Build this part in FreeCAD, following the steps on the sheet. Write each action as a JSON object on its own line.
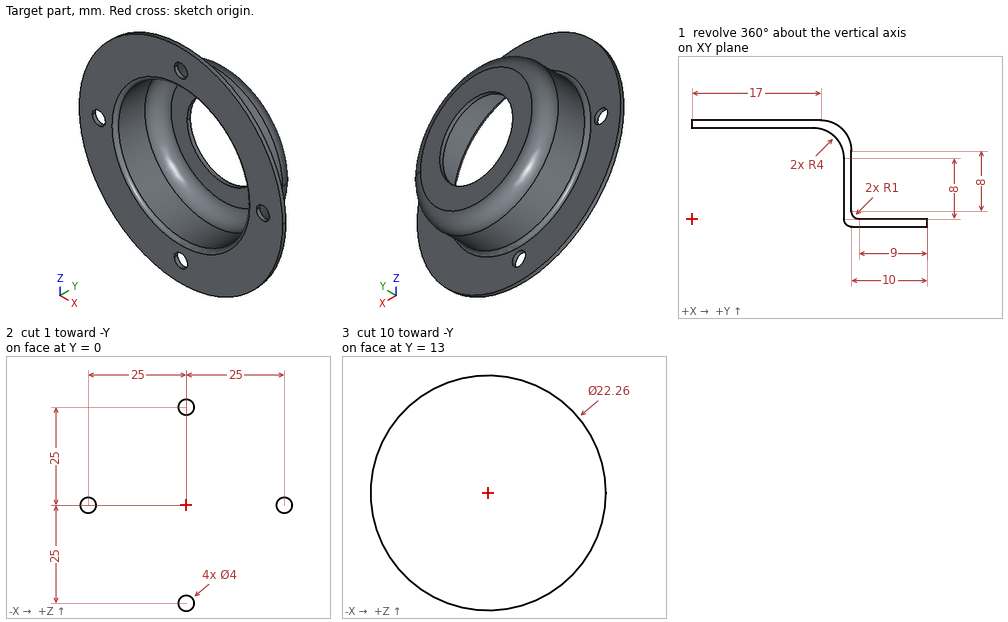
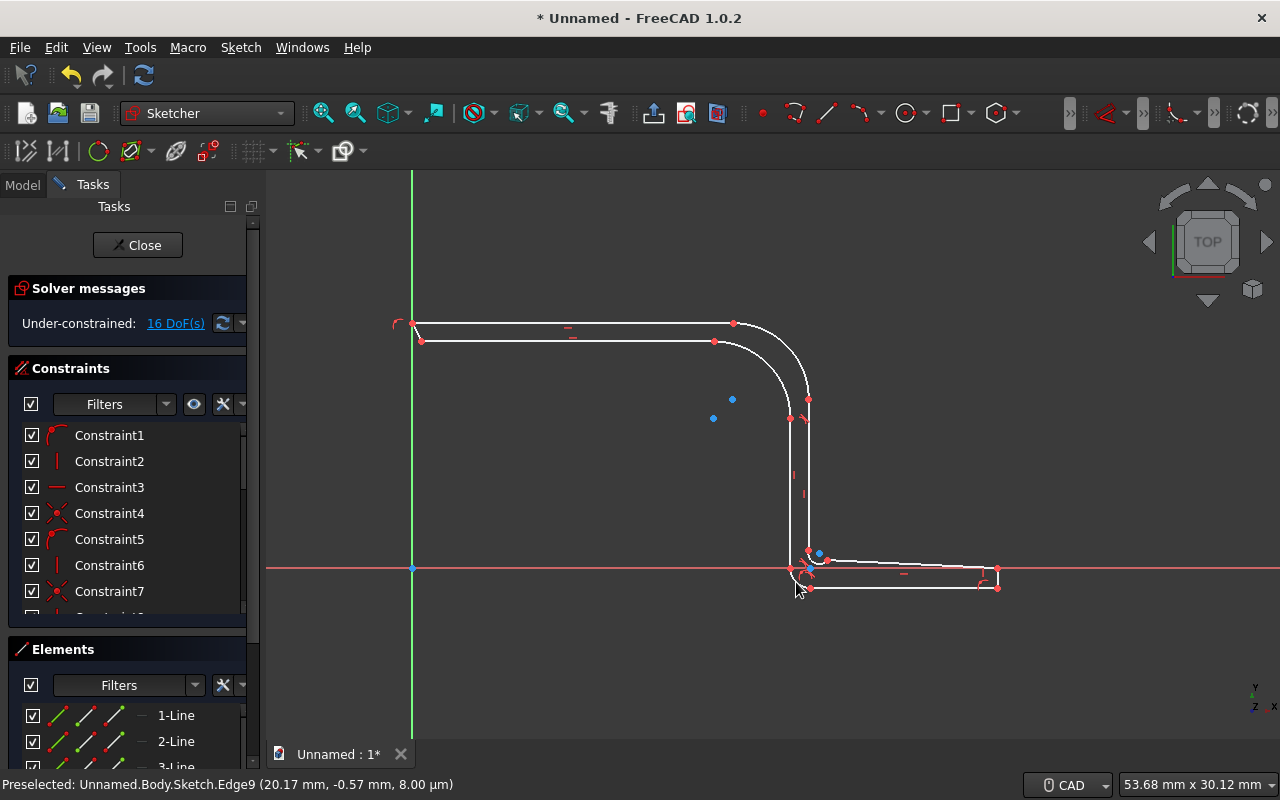
{"action": "left_click", "coordinate": [947, 566]}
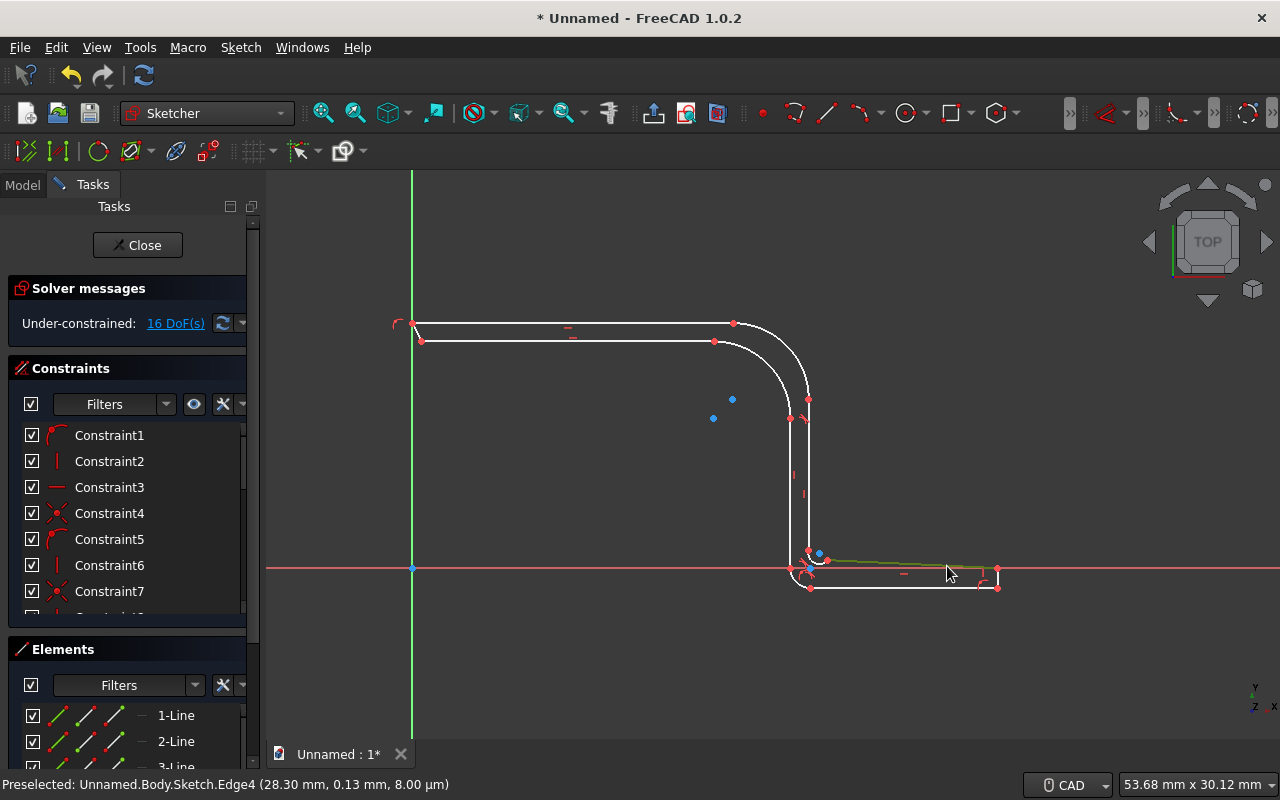
{"action": "scroll", "coordinate": [810, 559], "scroll_direction": "up", "scroll_amount": 3}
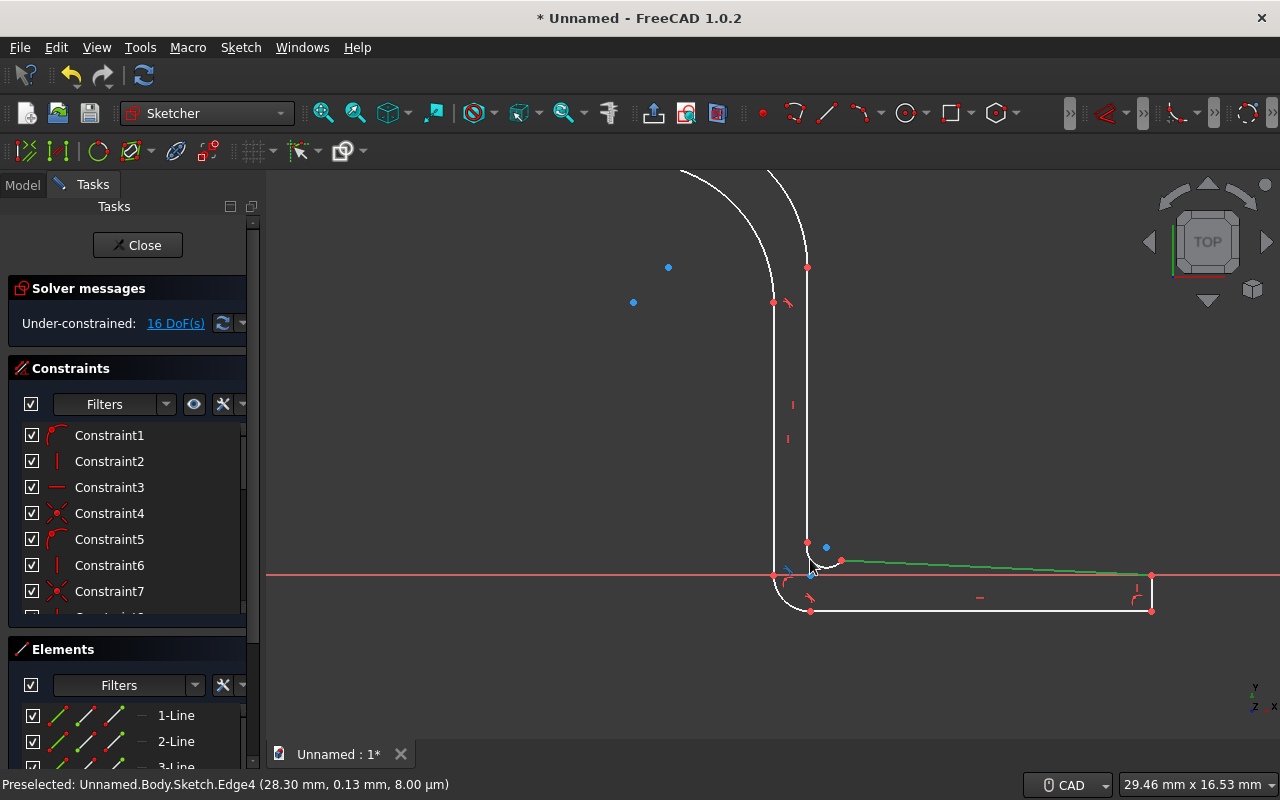
{"action": "left_click", "coordinate": [809, 558]}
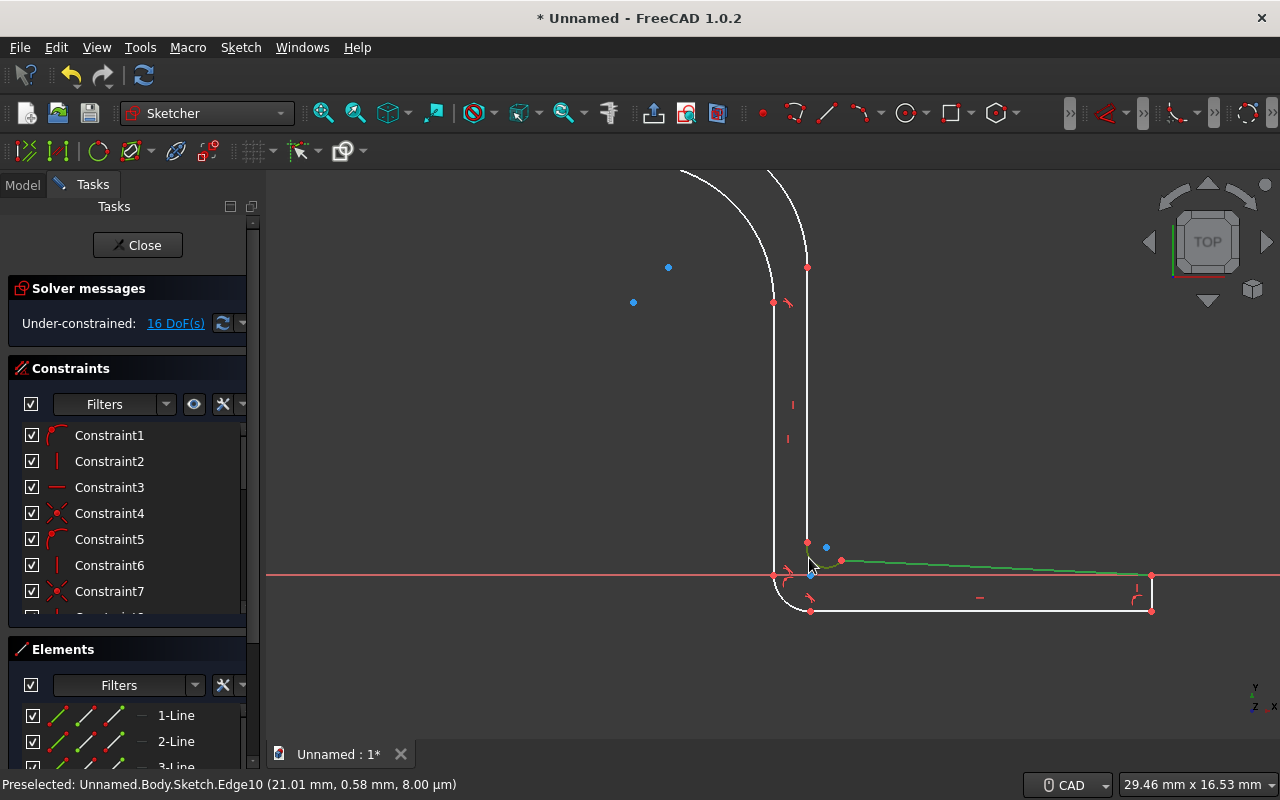
{"action": "key", "text": "t"}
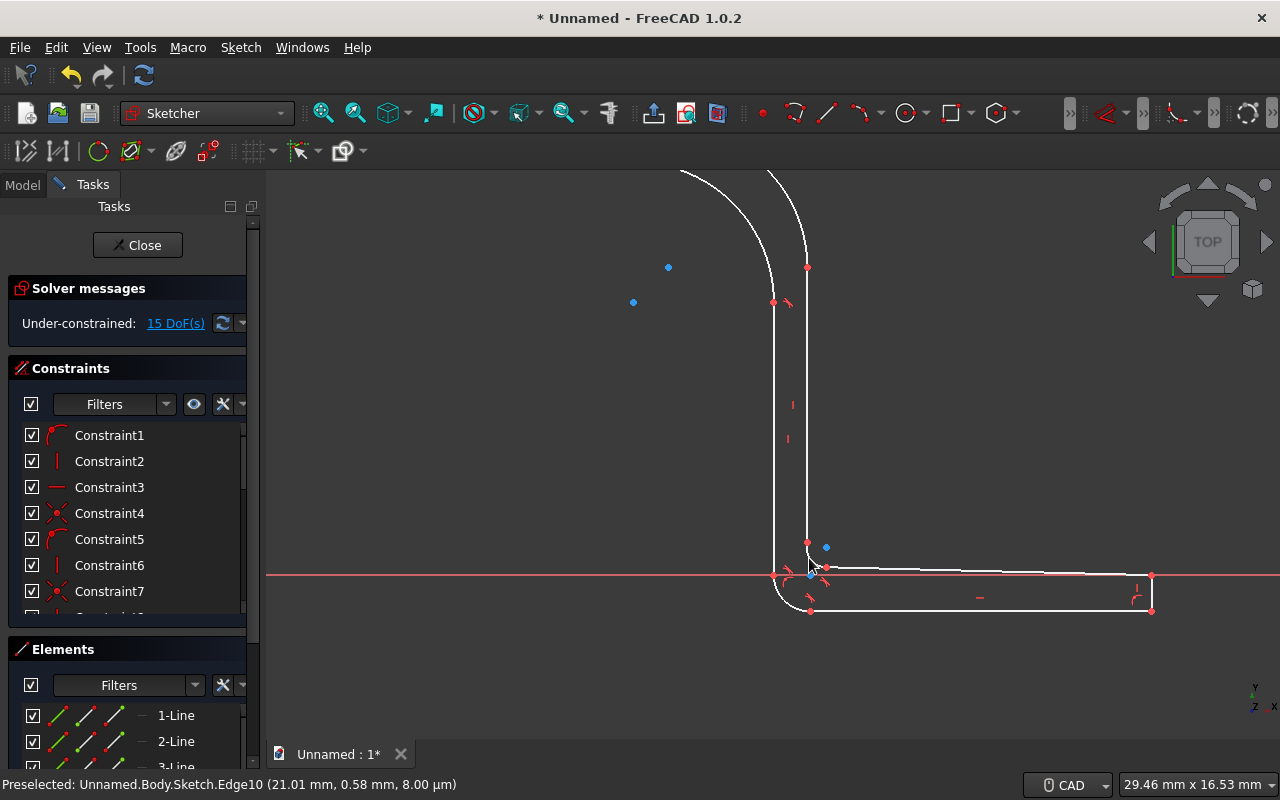
{"action": "left_click", "coordinate": [807, 460]}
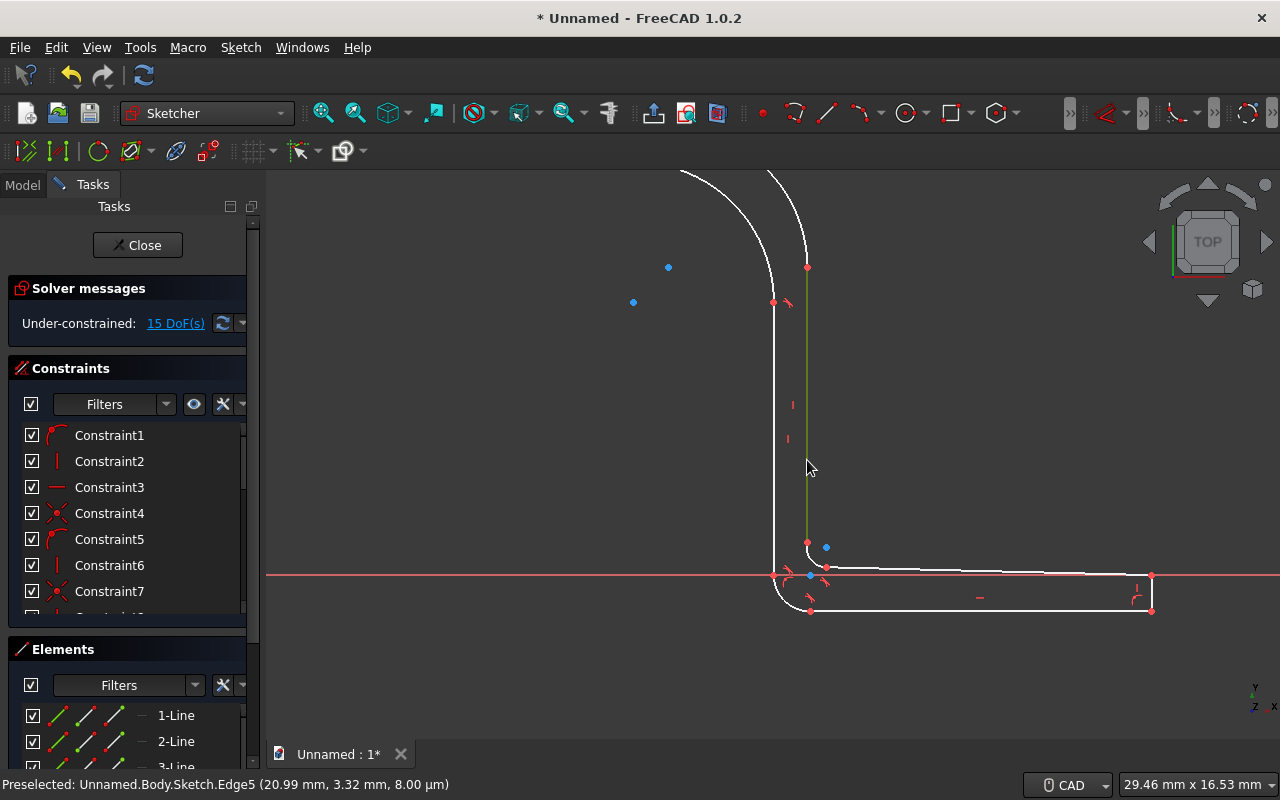
{"action": "scroll", "coordinate": [807, 553], "scroll_direction": "up", "scroll_amount": 2}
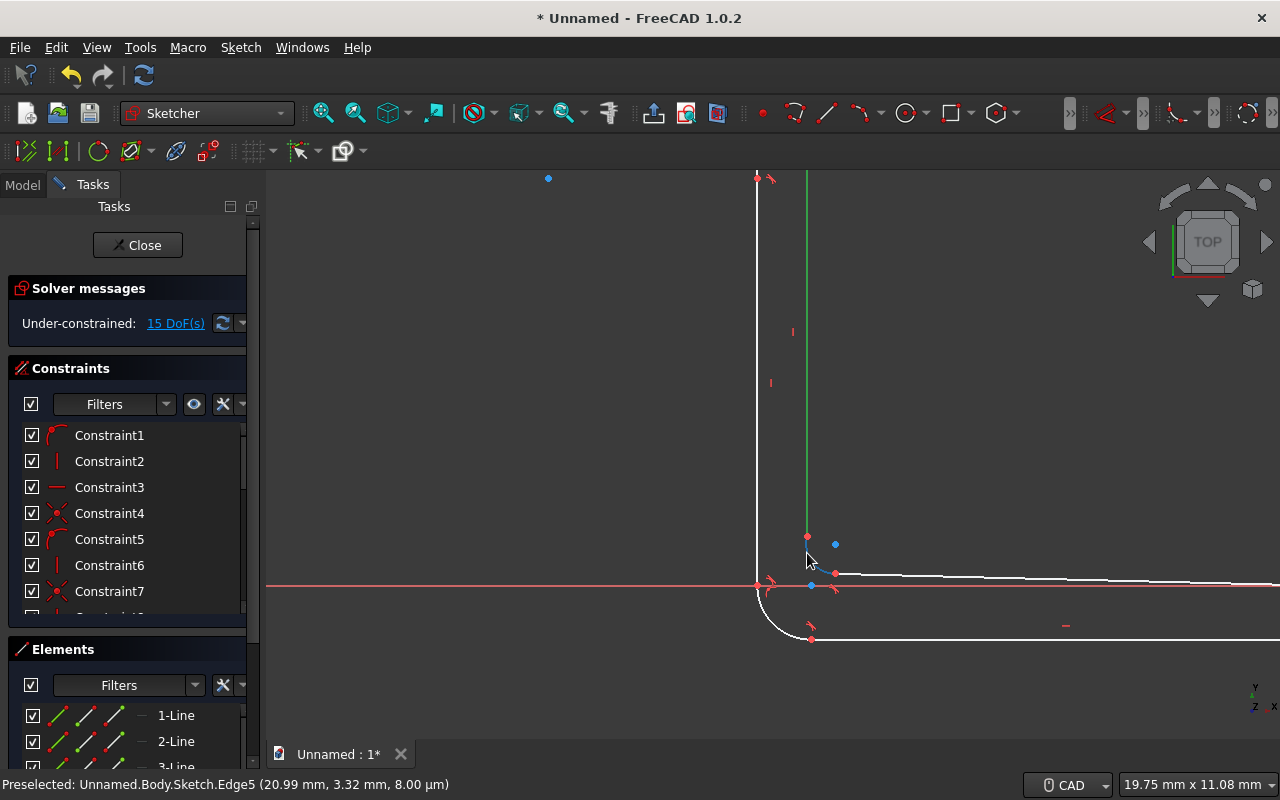
{"action": "left_click", "coordinate": [807, 552]}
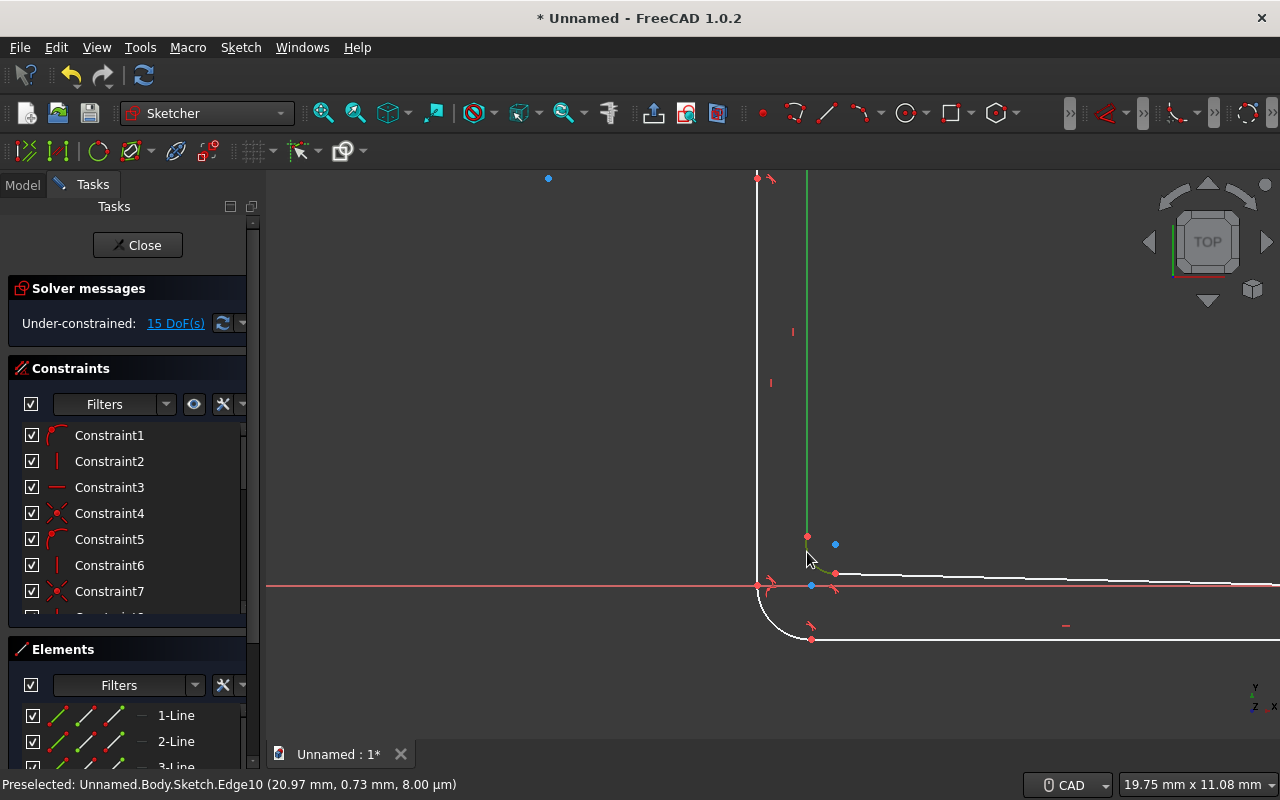
{"action": "key", "text": "t"}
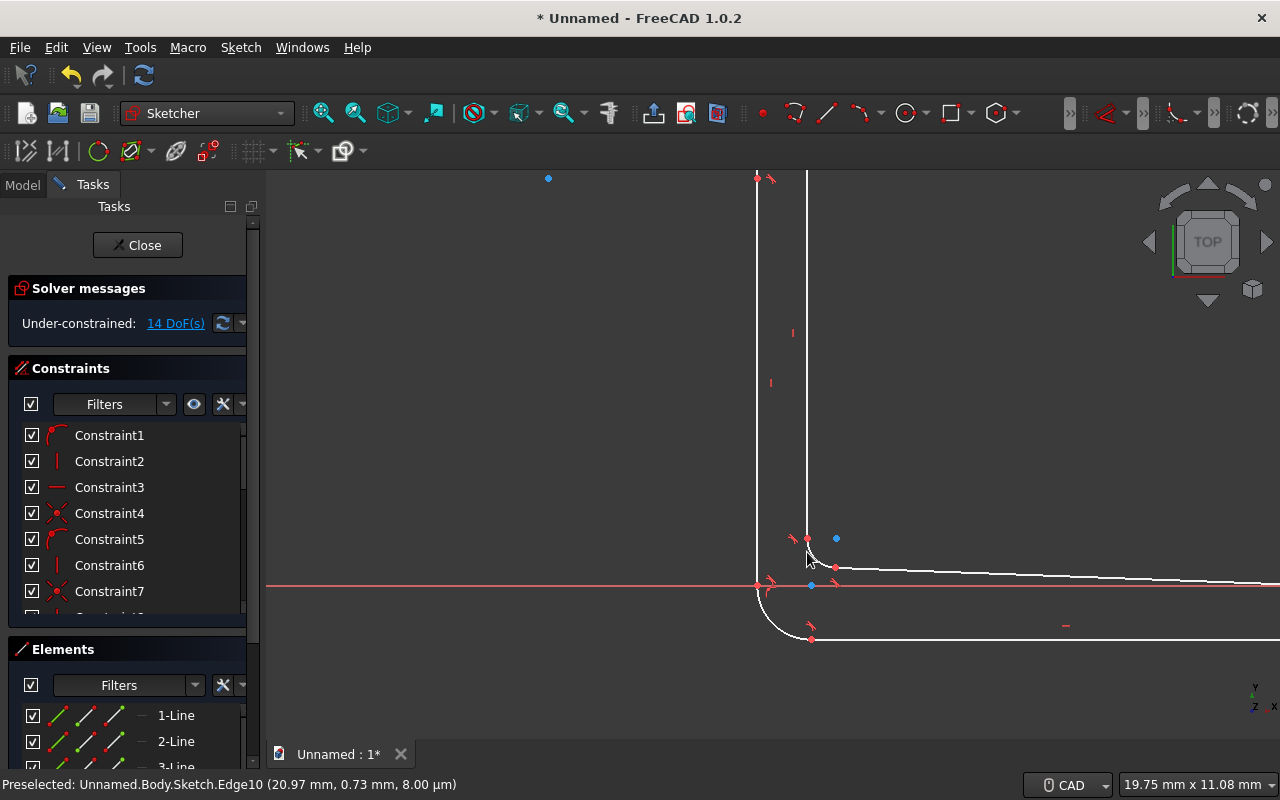
{"action": "left_click", "coordinate": [807, 415]}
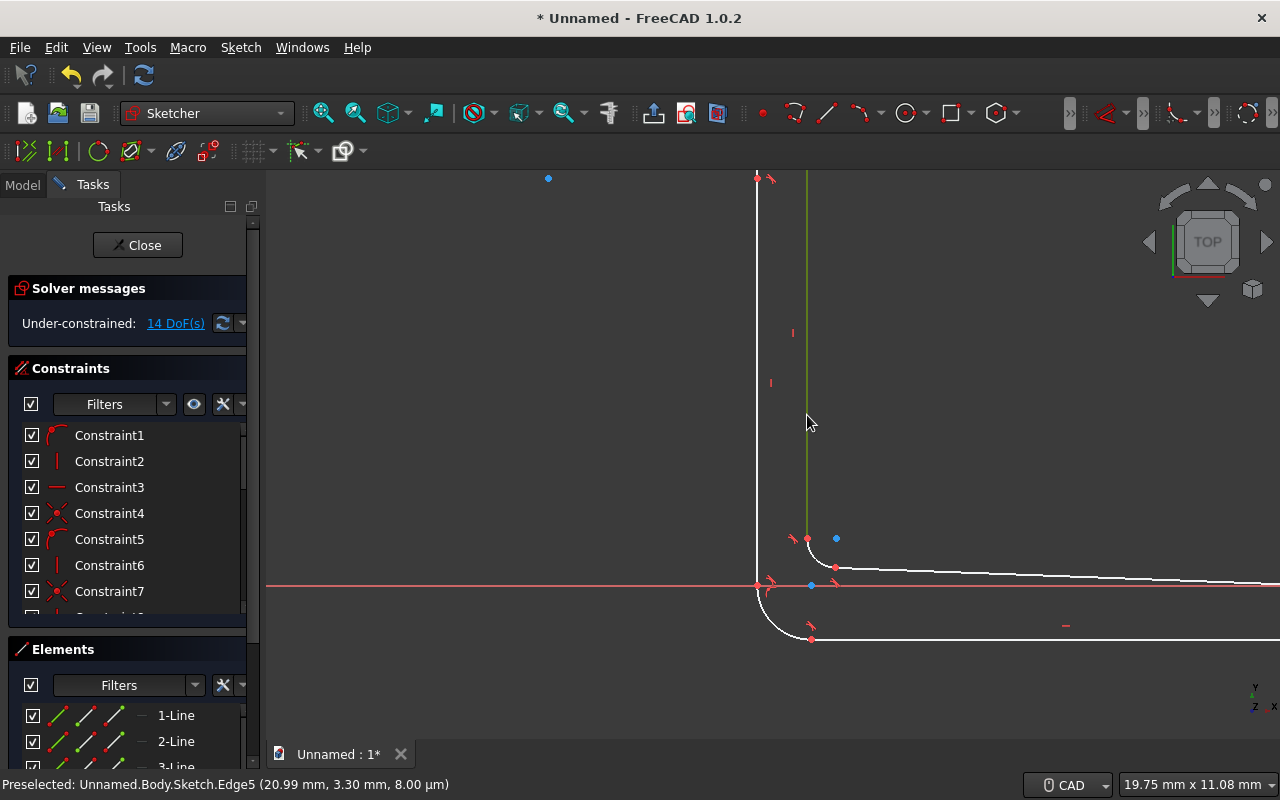
{"action": "scroll", "coordinate": [809, 557], "scroll_direction": "down", "scroll_amount": 5}